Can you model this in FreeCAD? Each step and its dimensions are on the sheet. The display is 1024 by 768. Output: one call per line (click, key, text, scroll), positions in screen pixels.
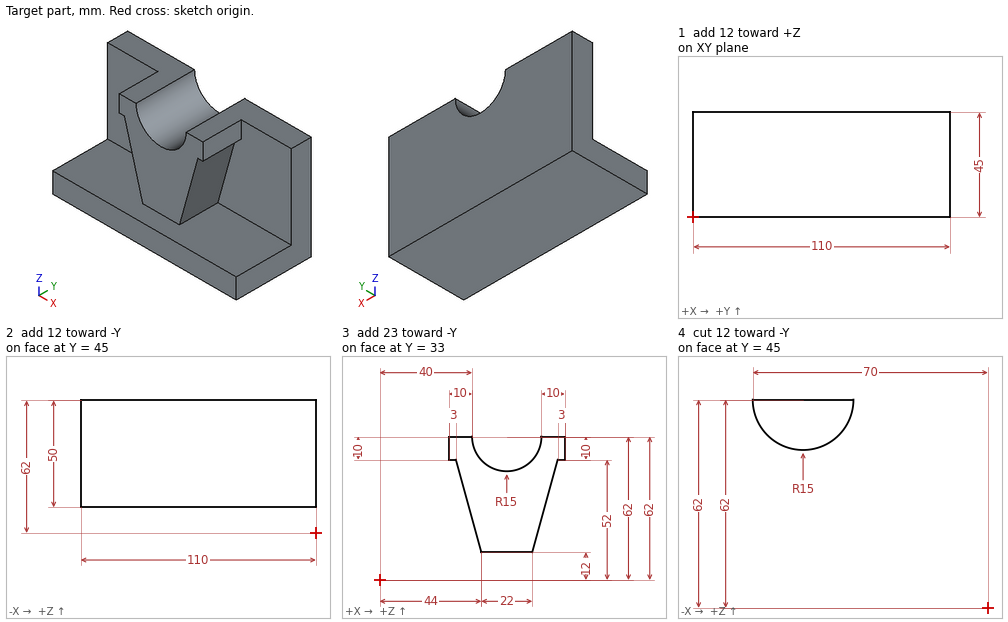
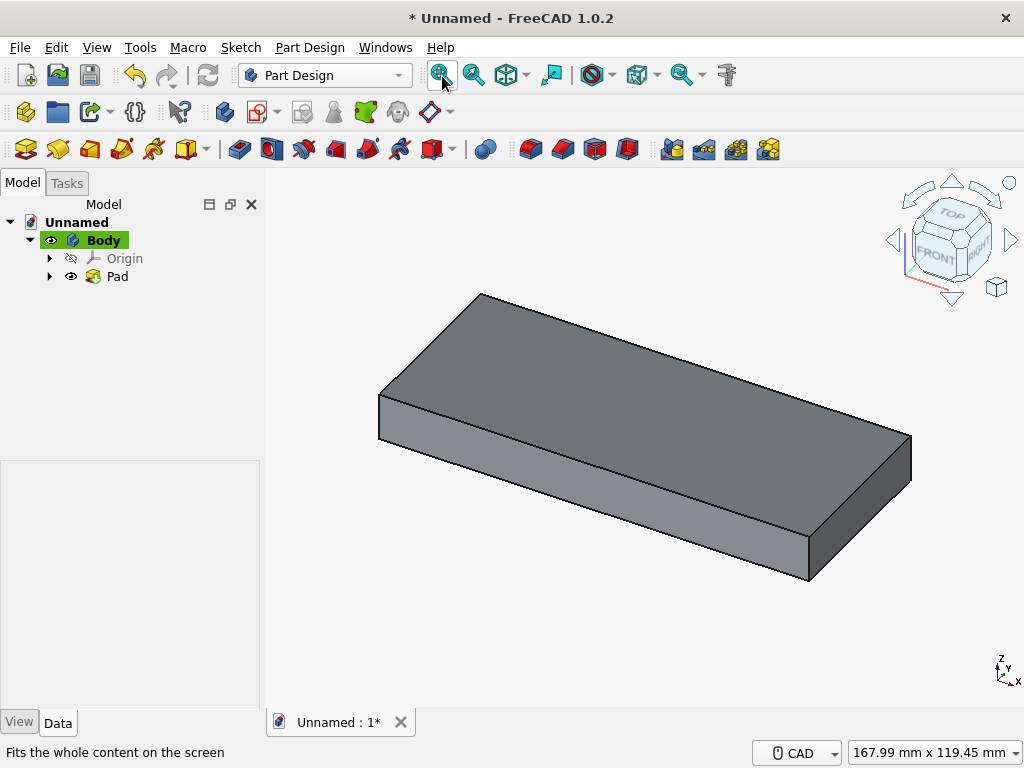
key(4)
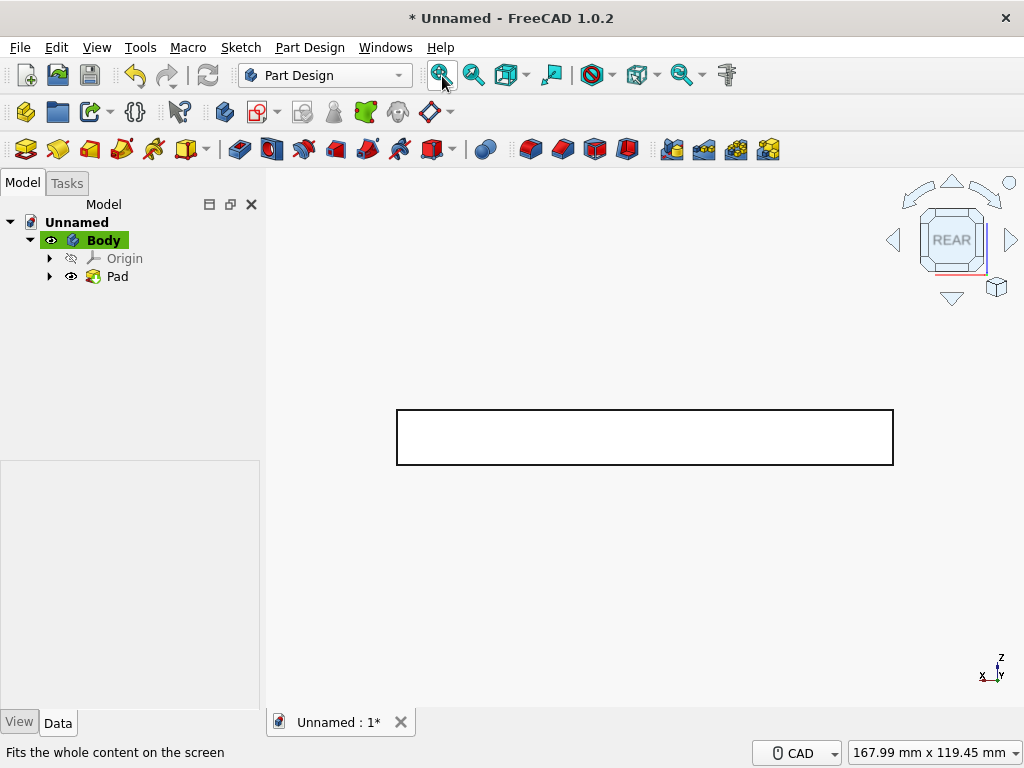
click(432, 437)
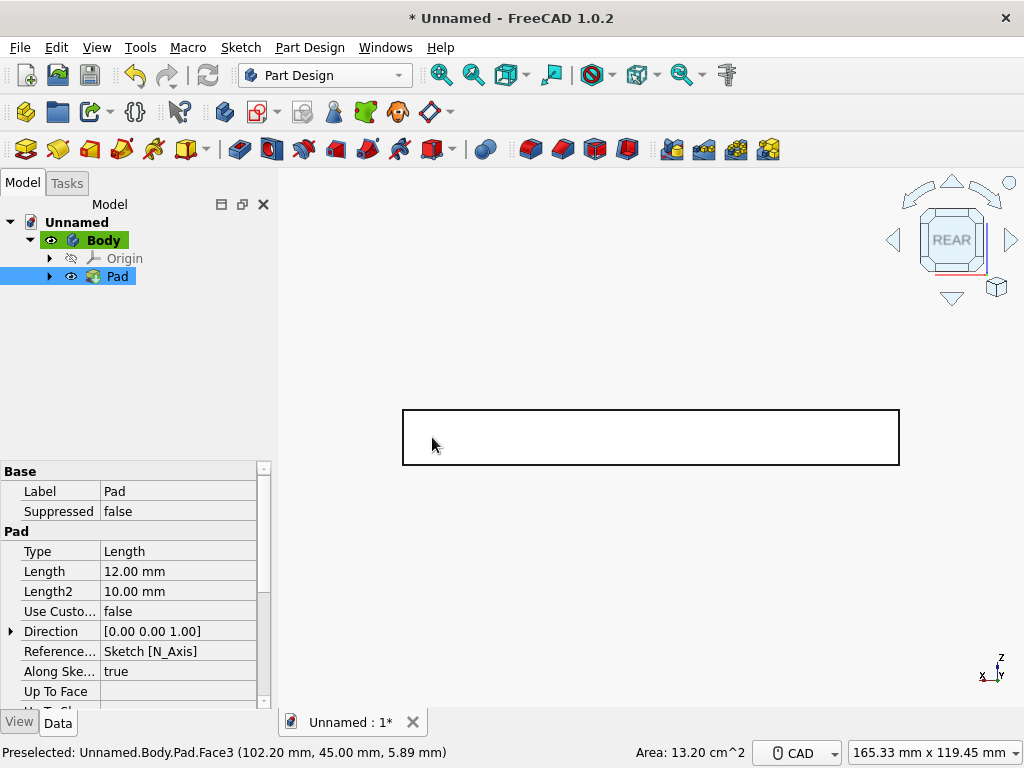
click(258, 112)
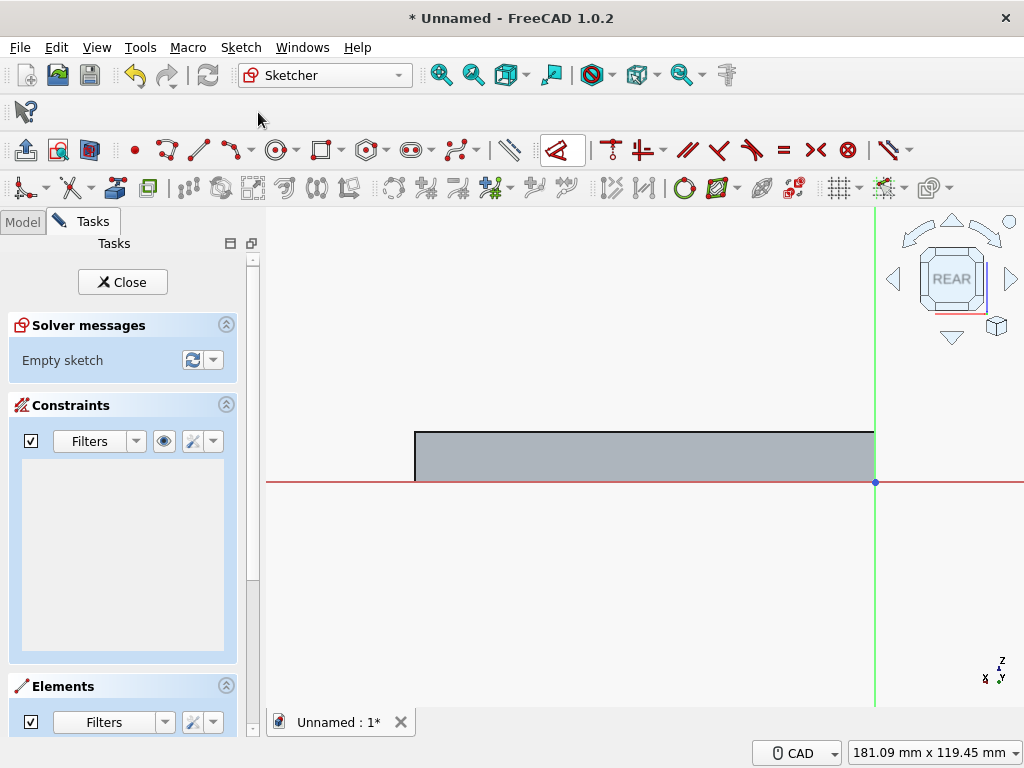
scroll(294, 679, down, 1)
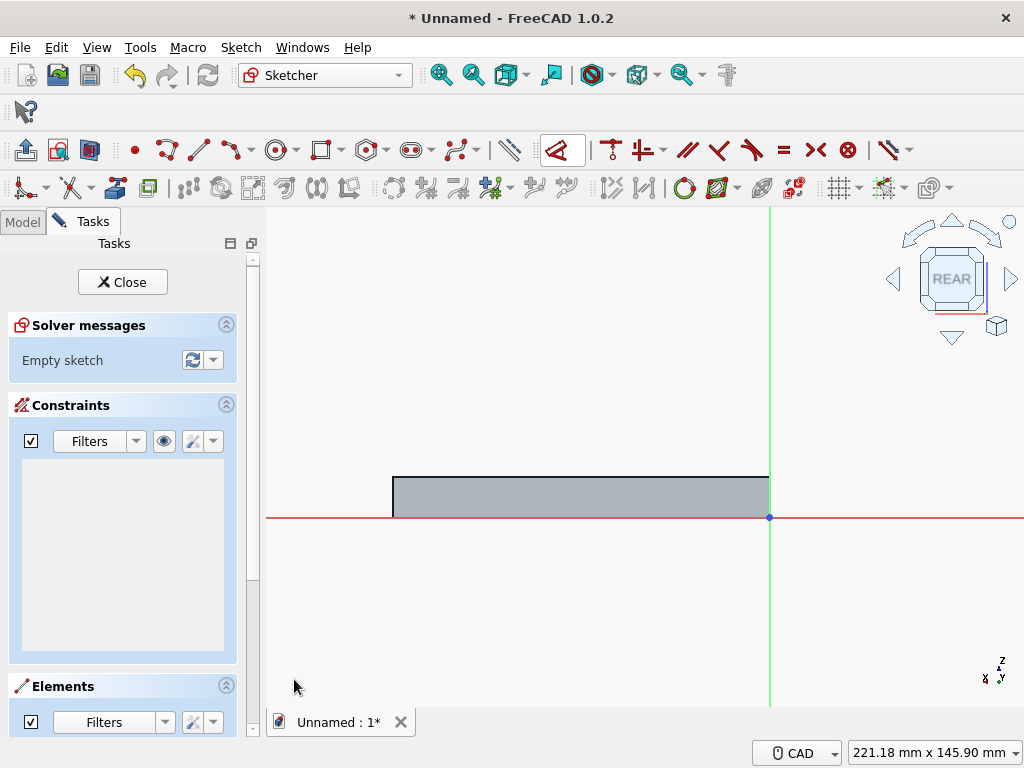
click(322, 150)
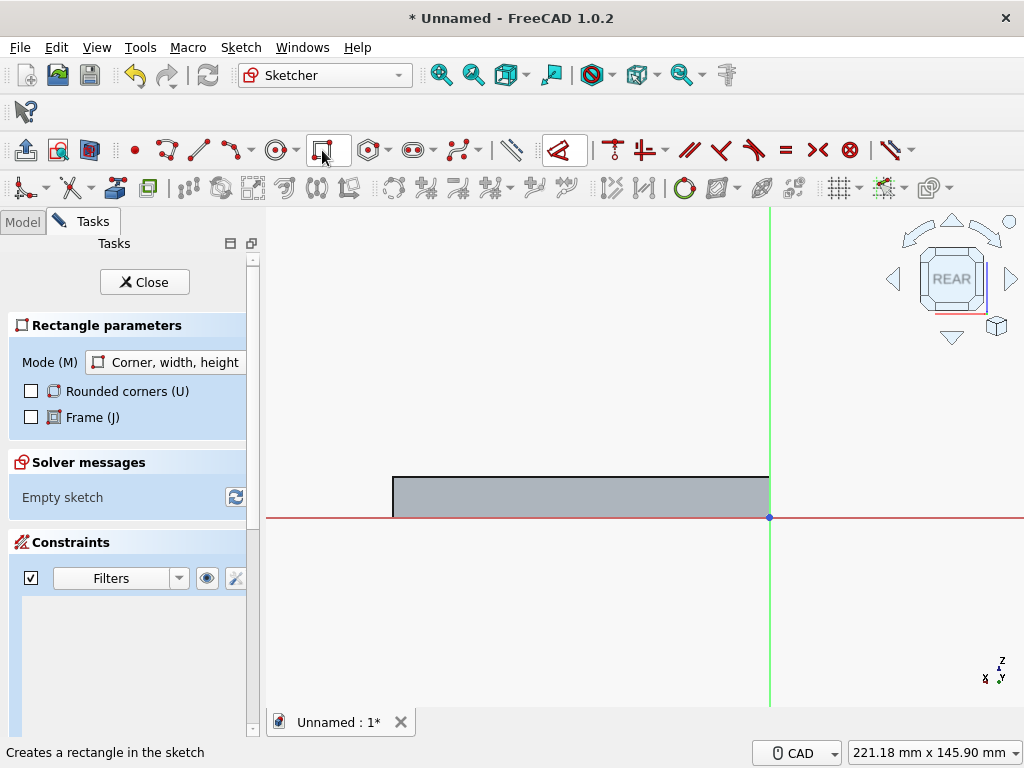
click(393, 306)
click(770, 477)
key(Escape)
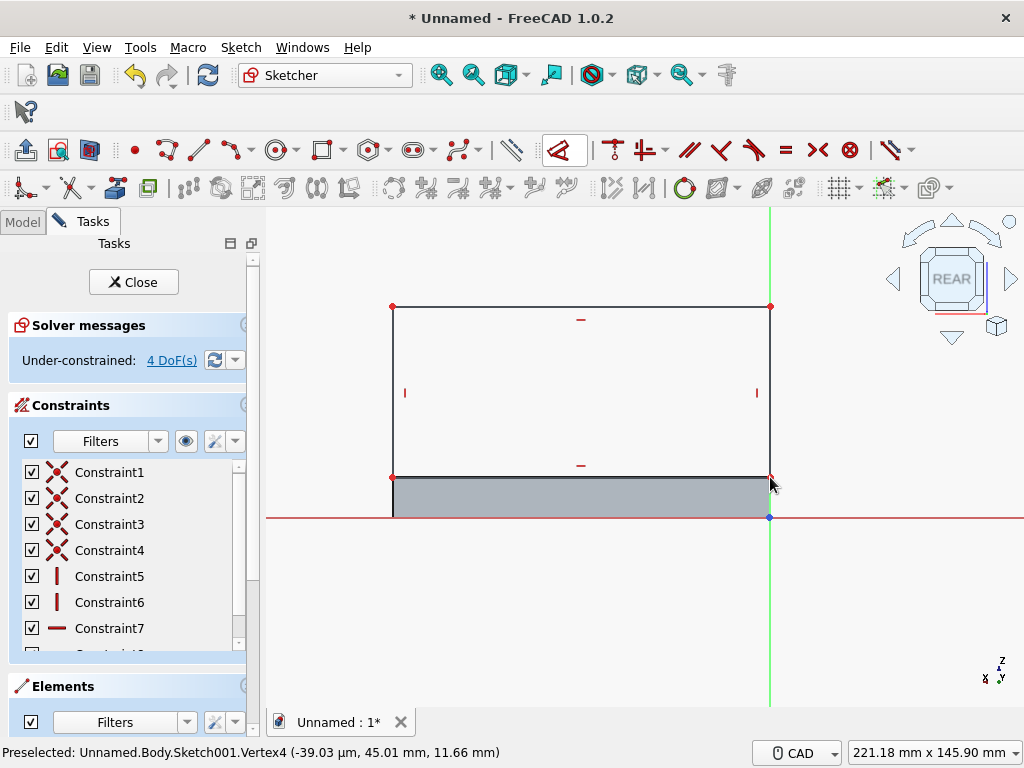
click(770, 478)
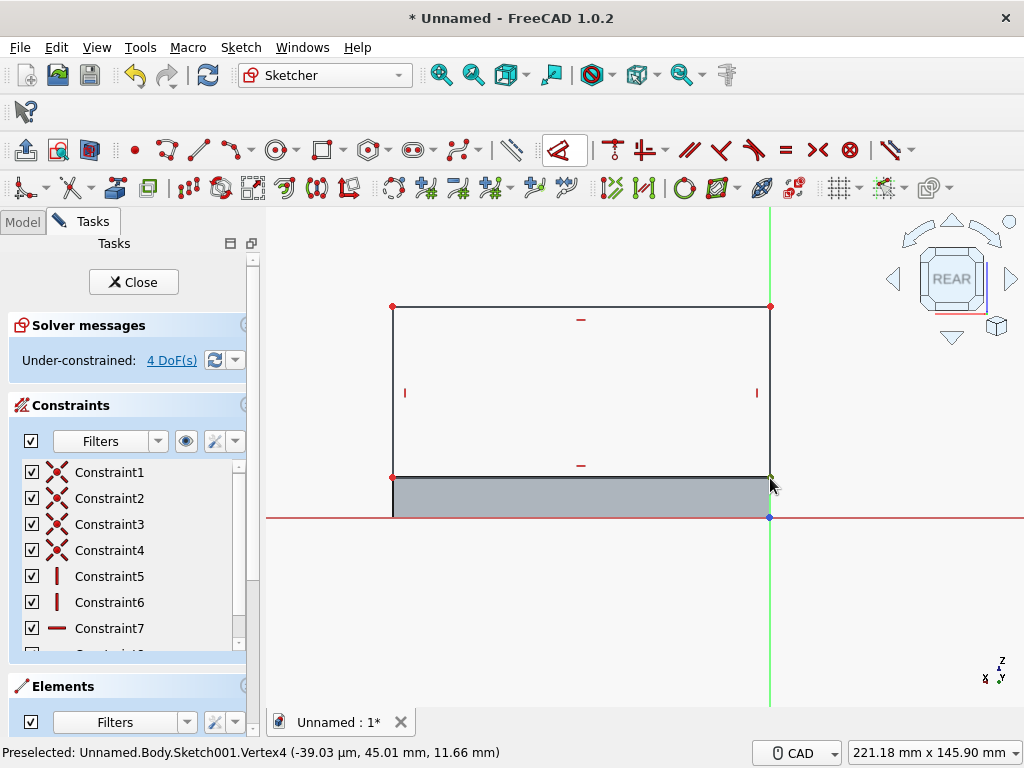
click(770, 647)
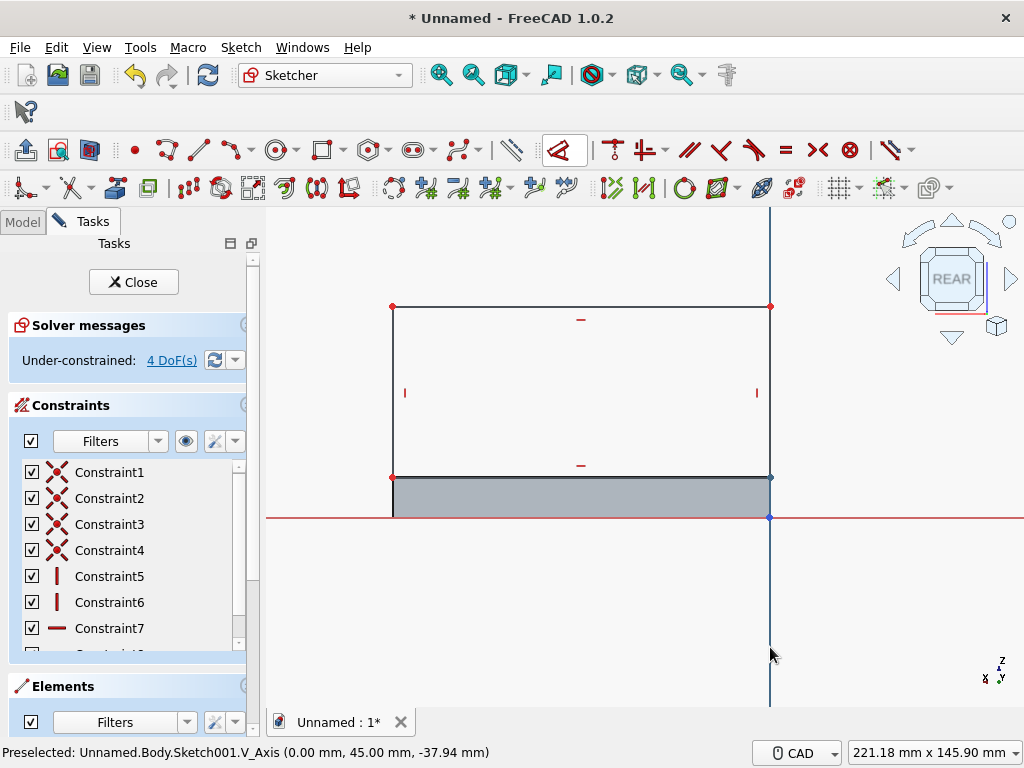
click(614, 150)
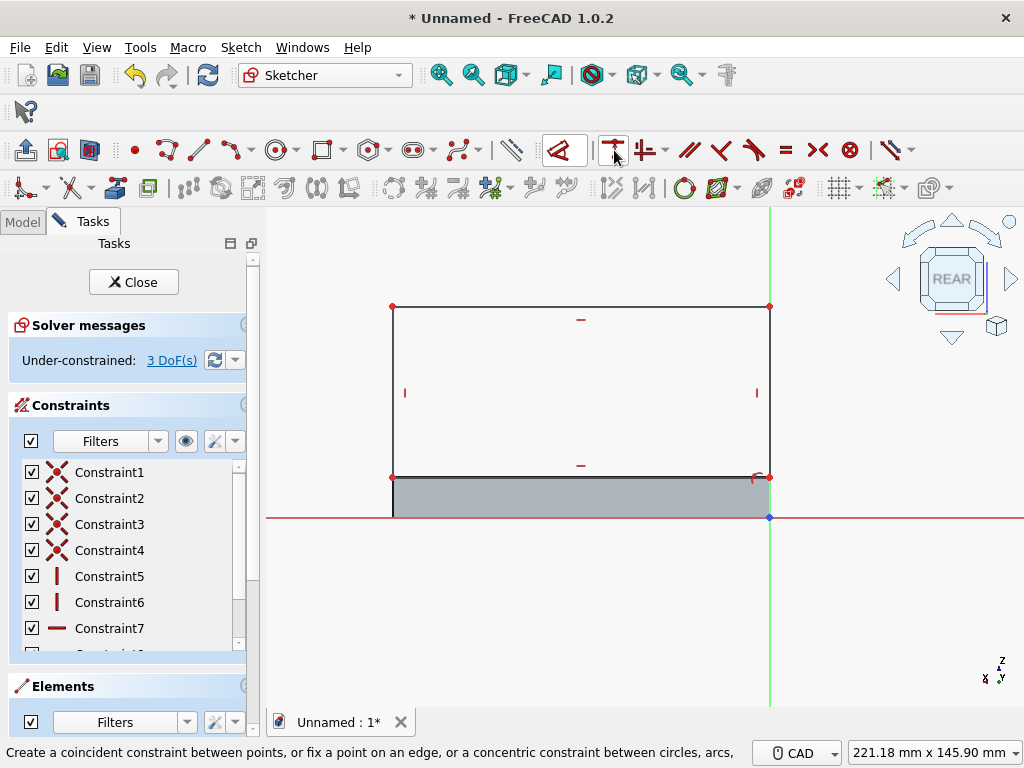
click(558, 150)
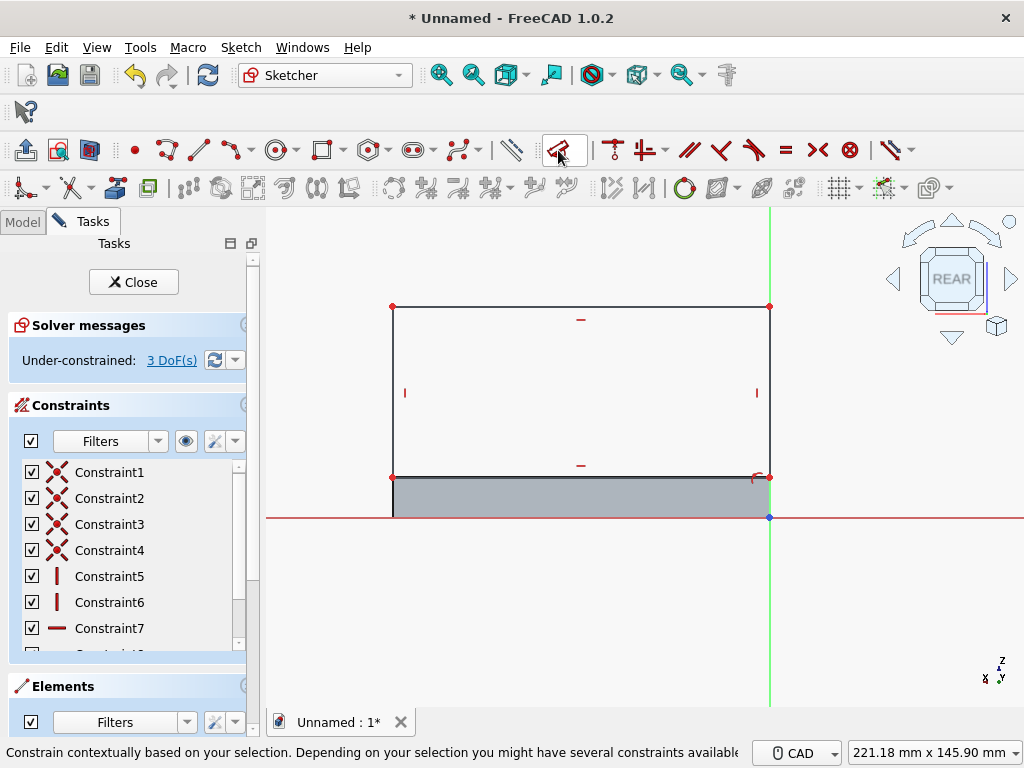
click(393, 358)
click(359, 392)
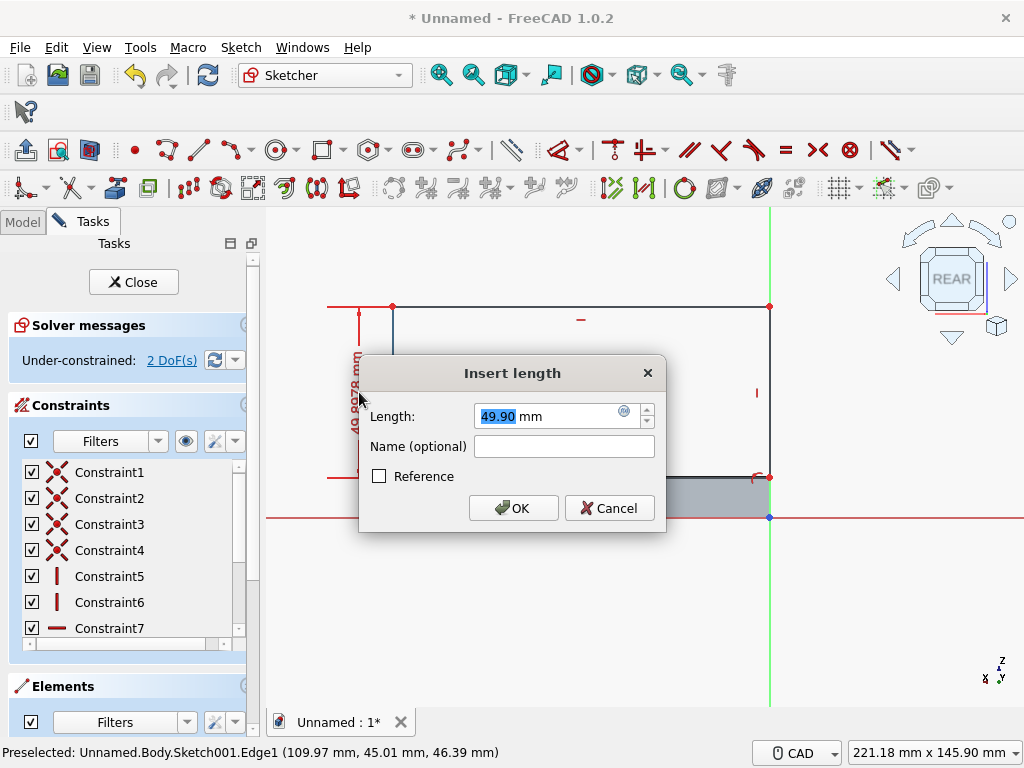
text(50)
key(Return)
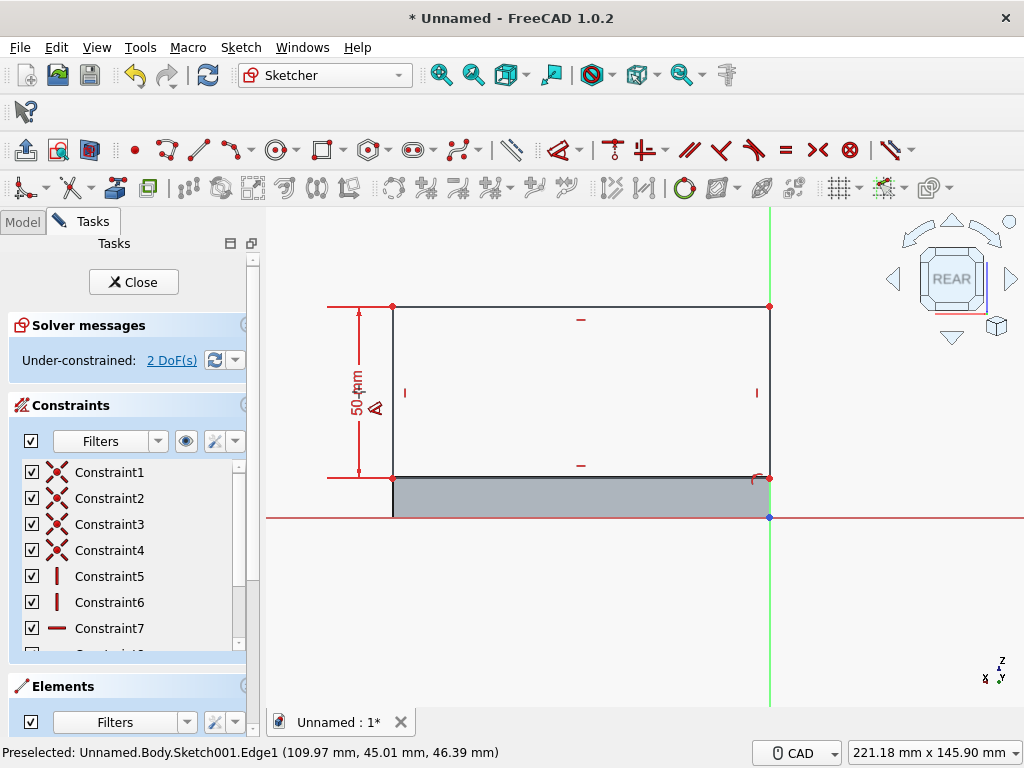
click(506, 478)
click(581, 444)